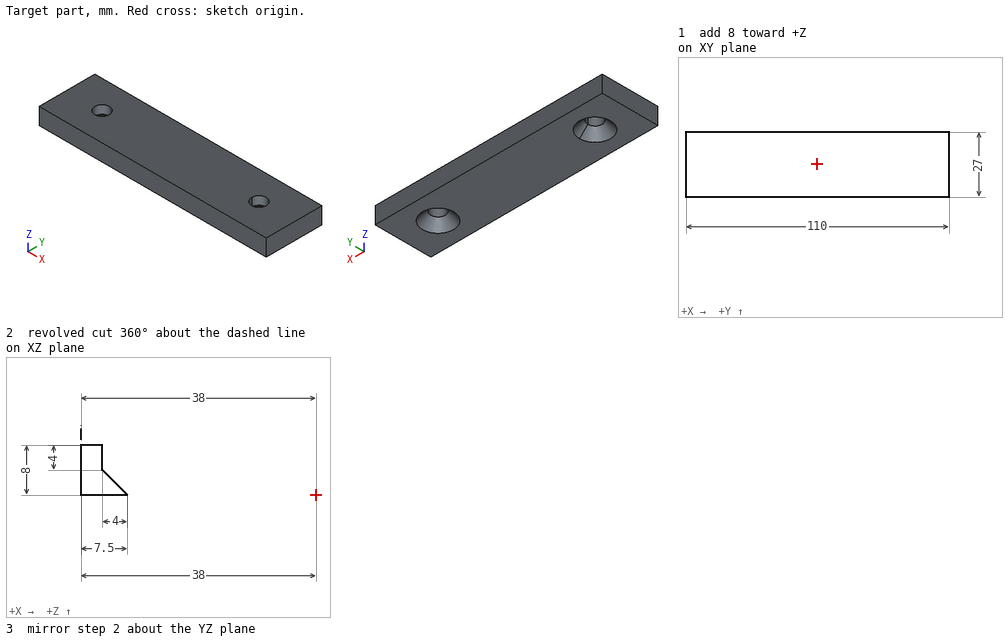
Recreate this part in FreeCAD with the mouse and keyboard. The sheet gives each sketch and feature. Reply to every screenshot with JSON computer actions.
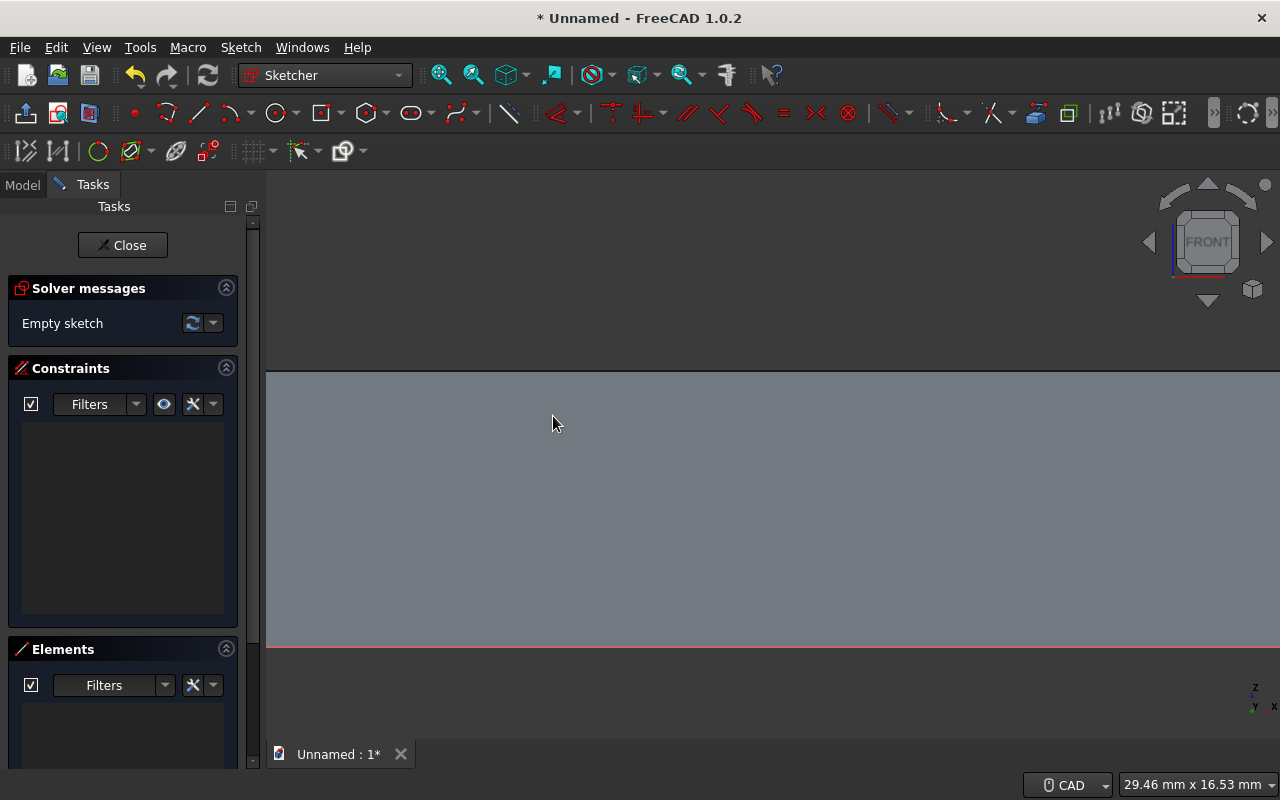
{"action": "left_click", "coordinate": [168, 114]}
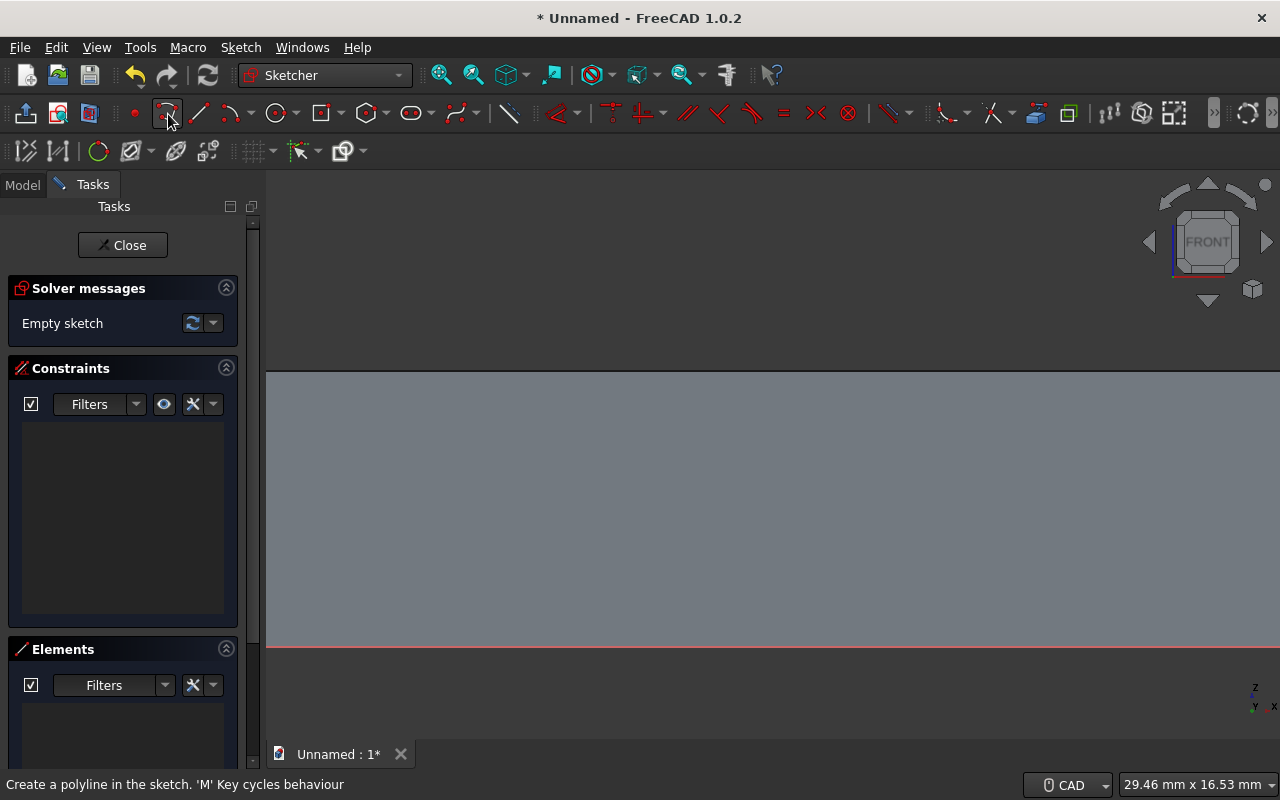
{"action": "left_click", "coordinate": [833, 647]}
{"action": "left_click", "coordinate": [574, 638]}
{"action": "left_click", "coordinate": [574, 371]}
{"action": "left_click", "coordinate": [695, 371]}
{"action": "left_click", "coordinate": [695, 509]}
{"action": "left_click", "coordinate": [833, 647]}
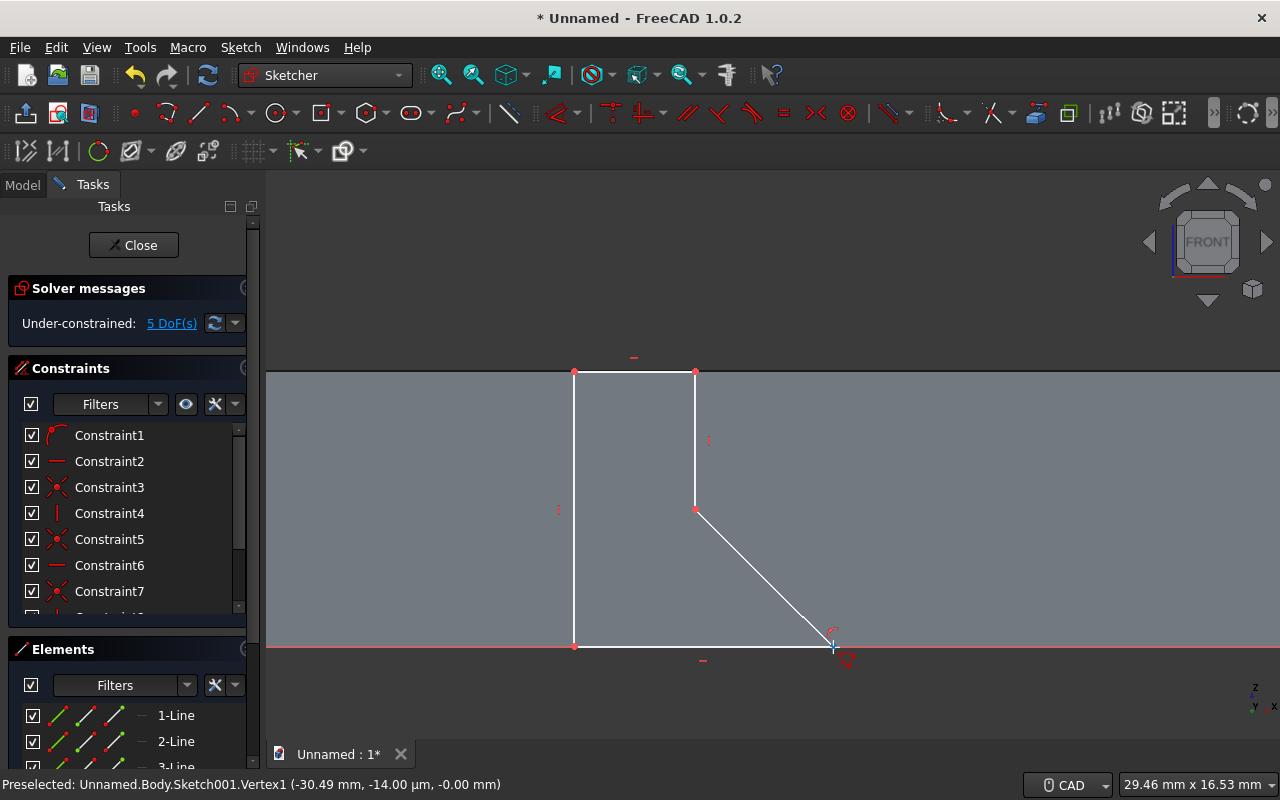
{"action": "left_click", "coordinate": [200, 114]}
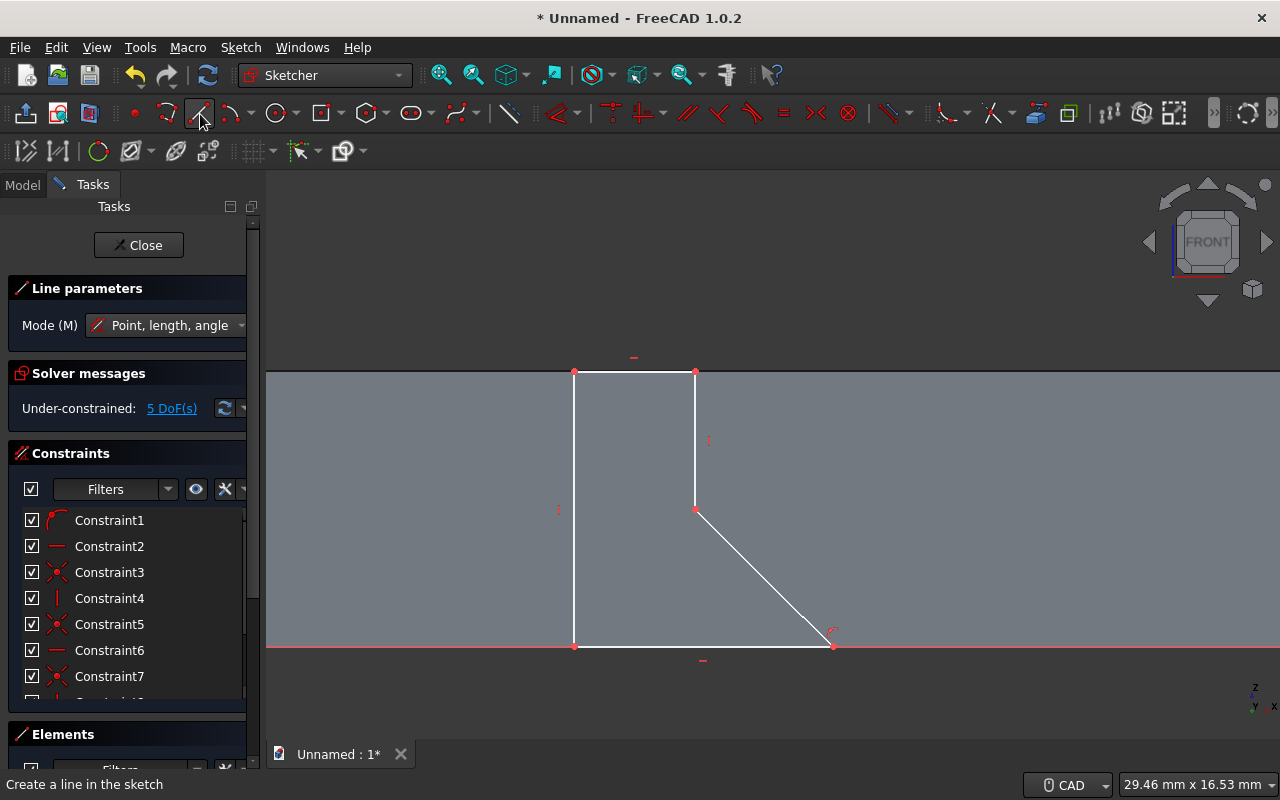
{"action": "left_click", "coordinate": [574, 344]}
{"action": "left_click", "coordinate": [574, 261]}
{"action": "key", "text": "Escape"}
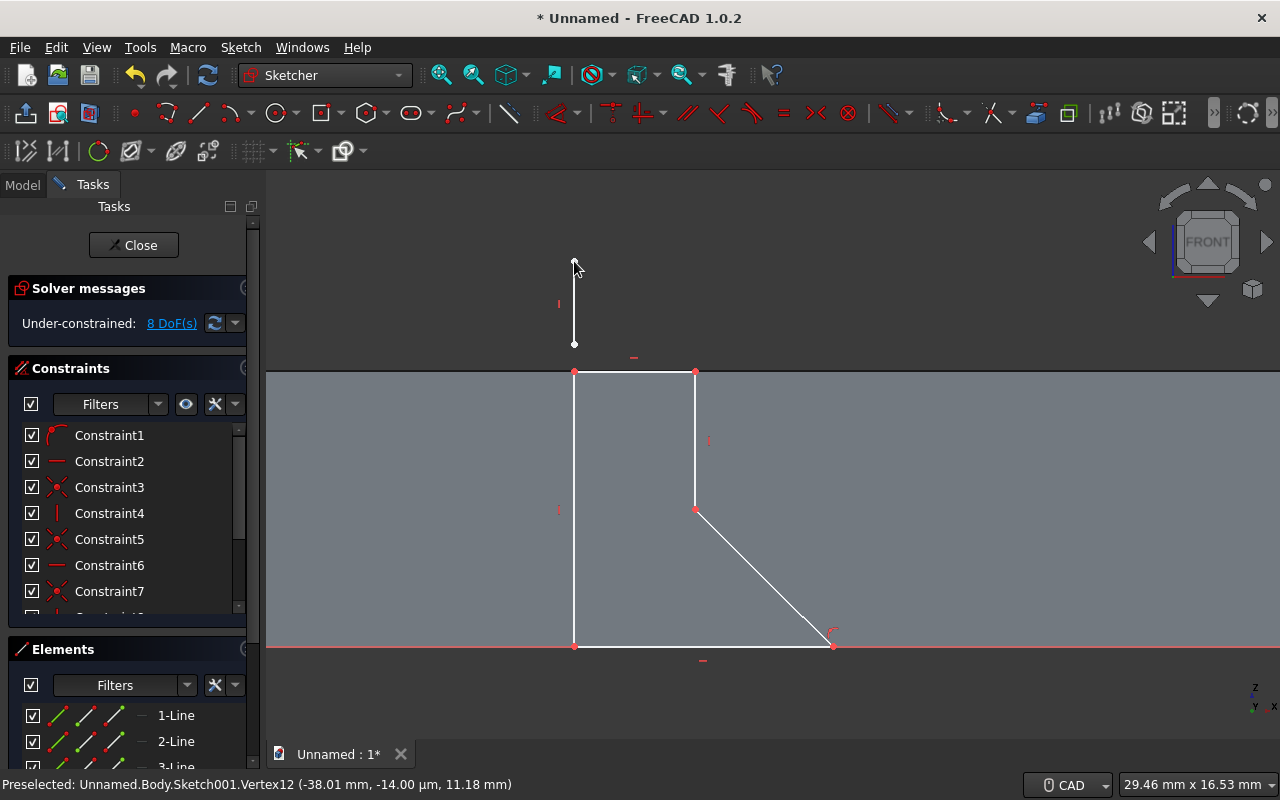
{"action": "left_click", "coordinate": [574, 320]}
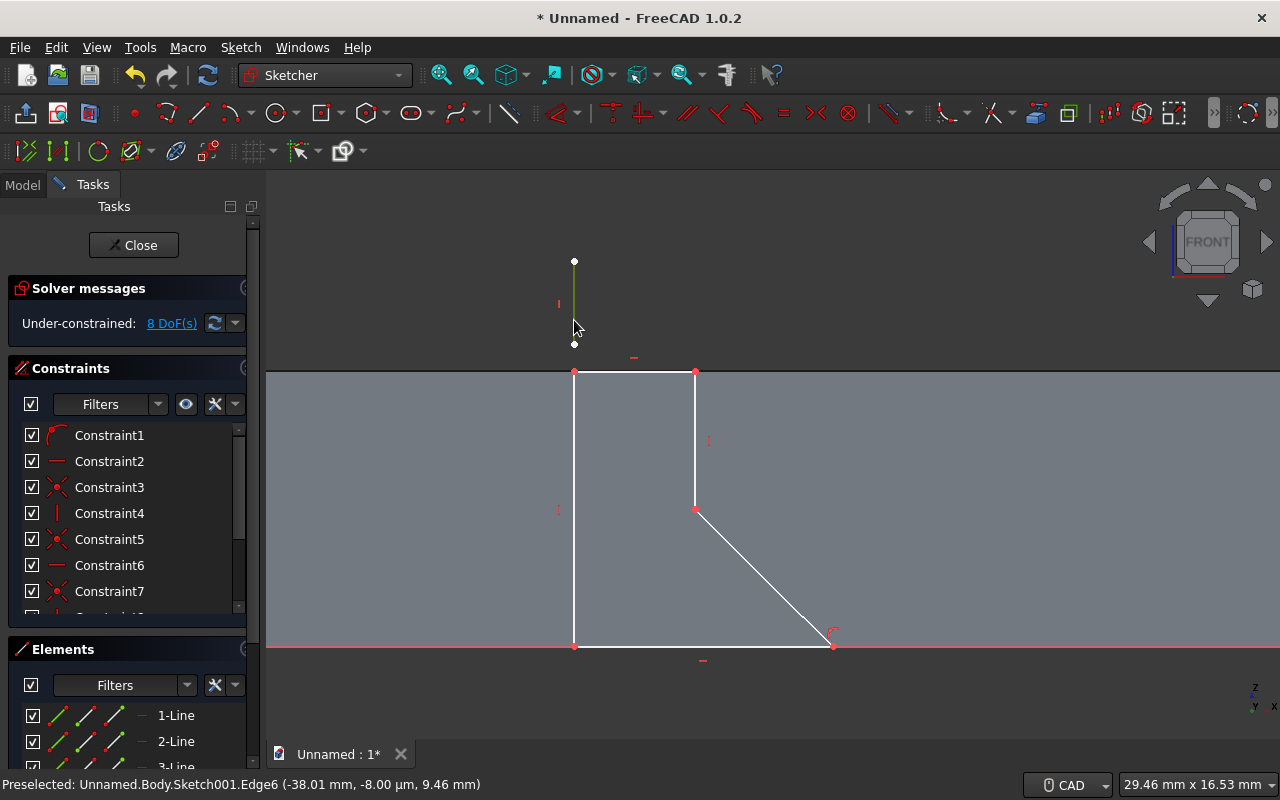
{"action": "left_click", "coordinate": [510, 114]}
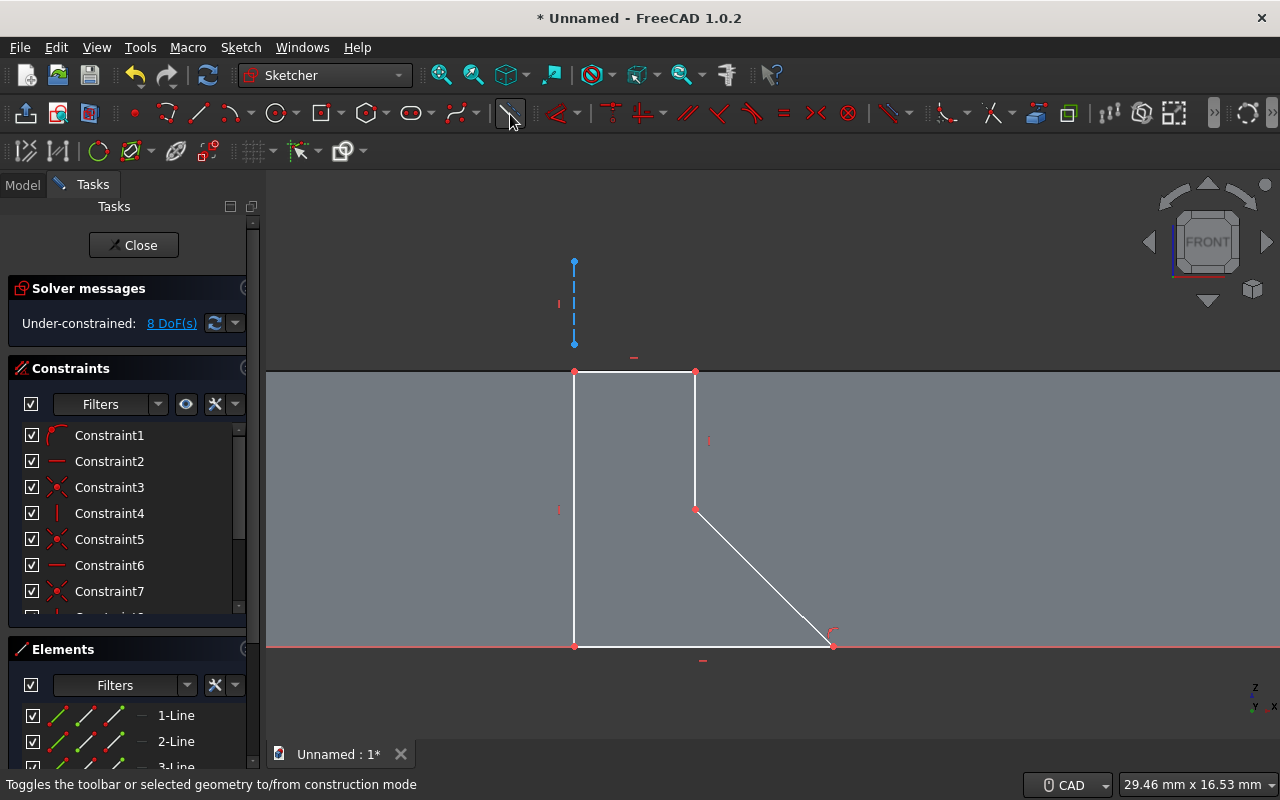
{"action": "left_click", "coordinate": [556, 114]}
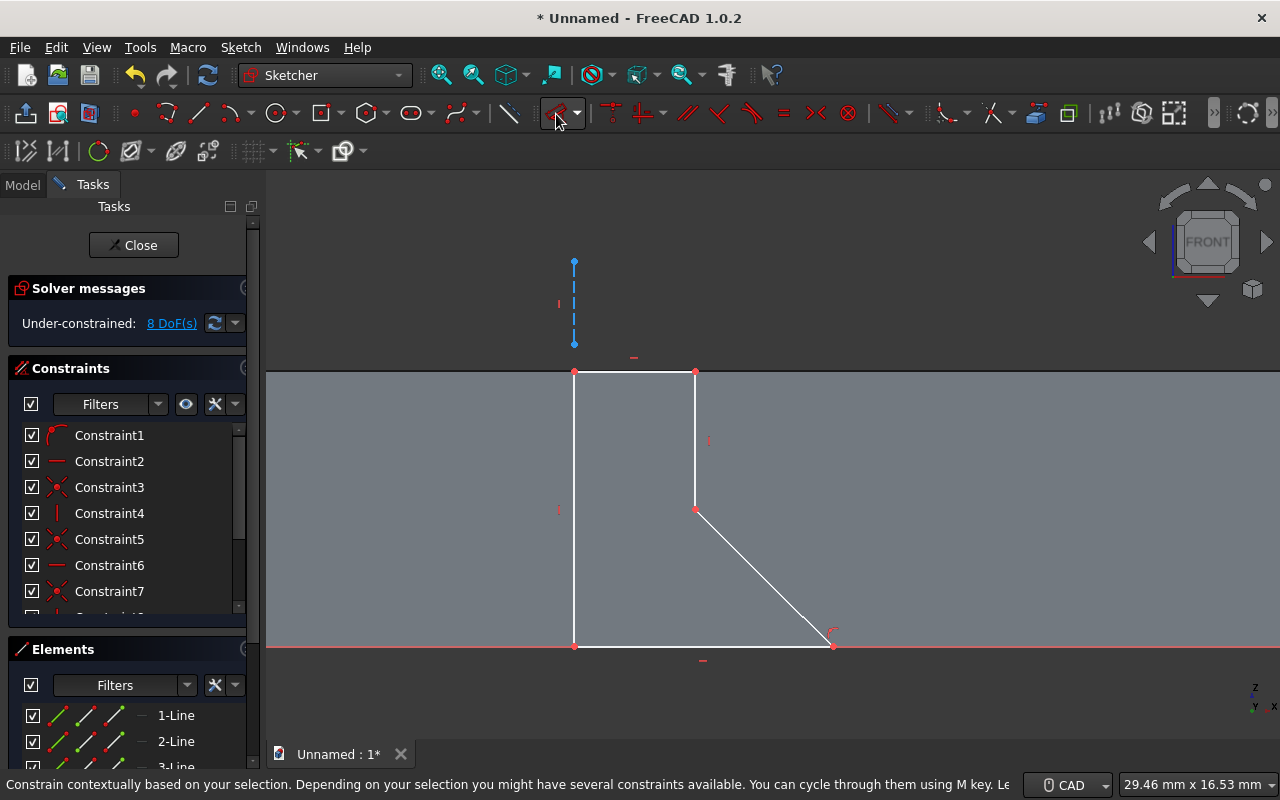
{"action": "left_click", "coordinate": [574, 564]}
{"action": "left_click", "coordinate": [540, 509]}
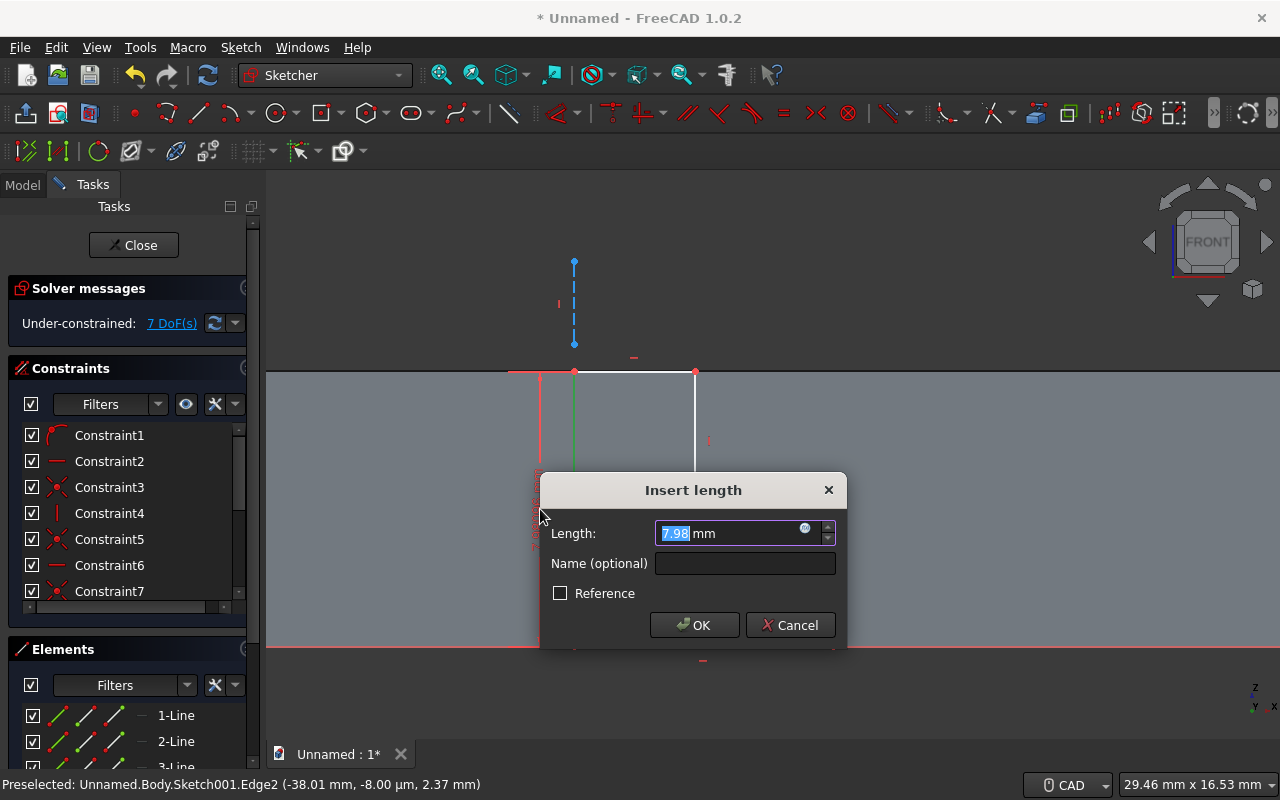
{"action": "type", "text": "8"}
{"action": "key", "text": "Return"}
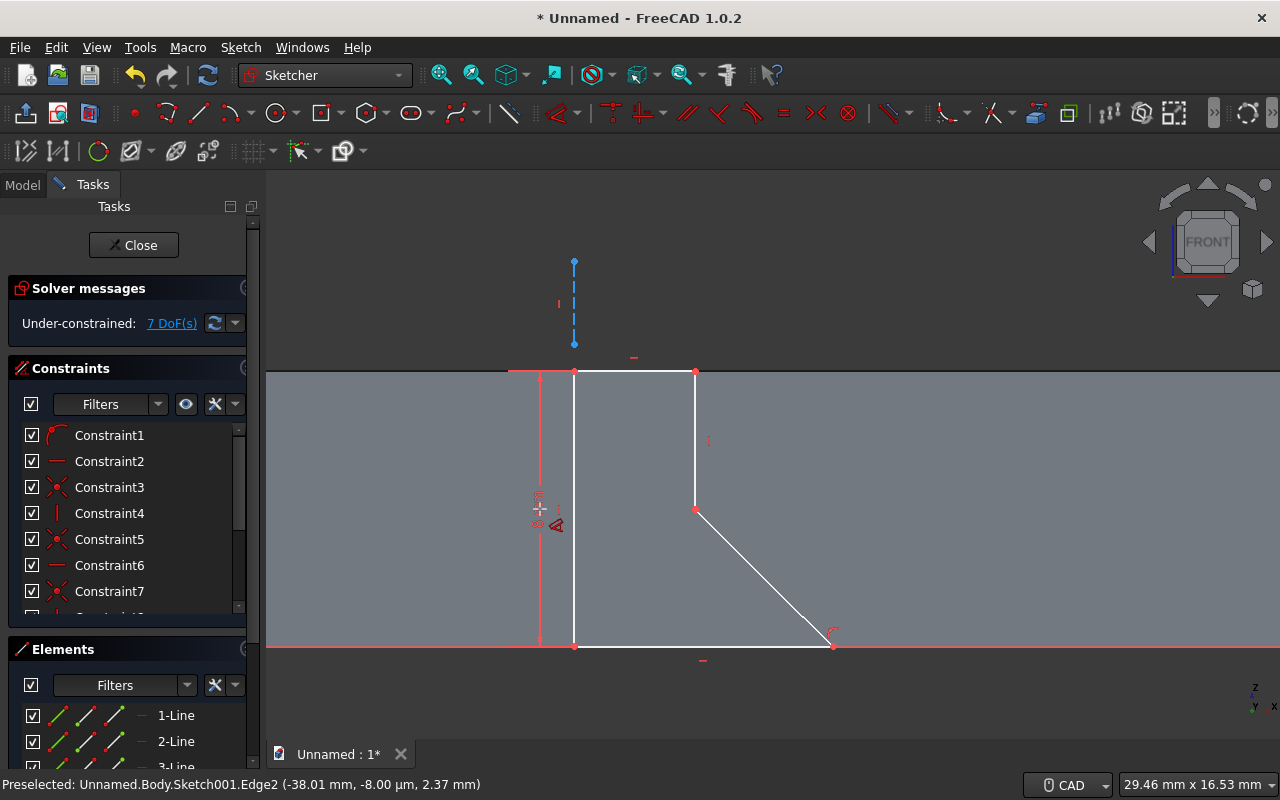
{"action": "left_click", "coordinate": [695, 413]}
{"action": "left_click", "coordinate": [661, 441]}